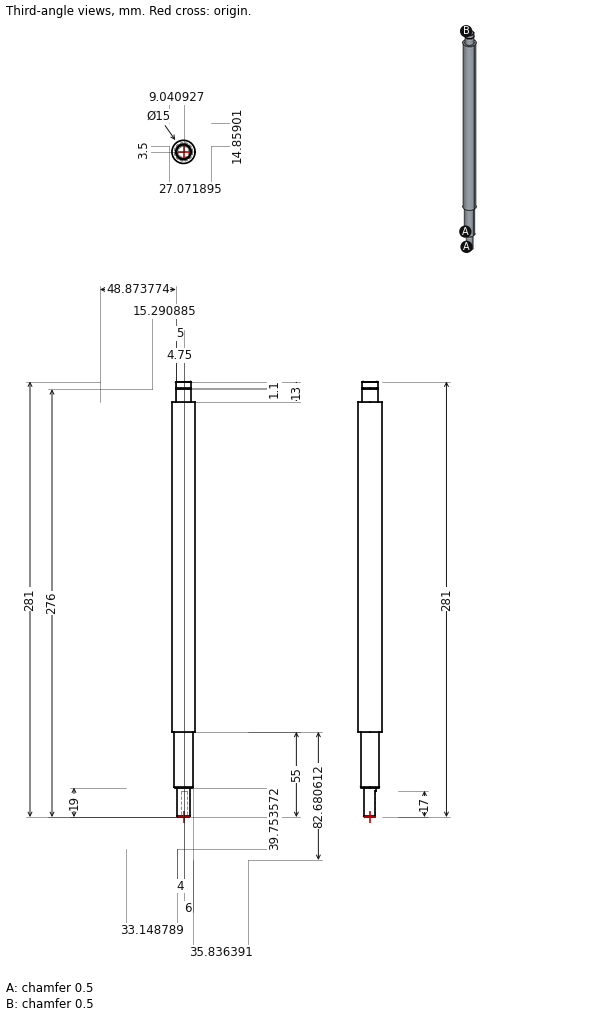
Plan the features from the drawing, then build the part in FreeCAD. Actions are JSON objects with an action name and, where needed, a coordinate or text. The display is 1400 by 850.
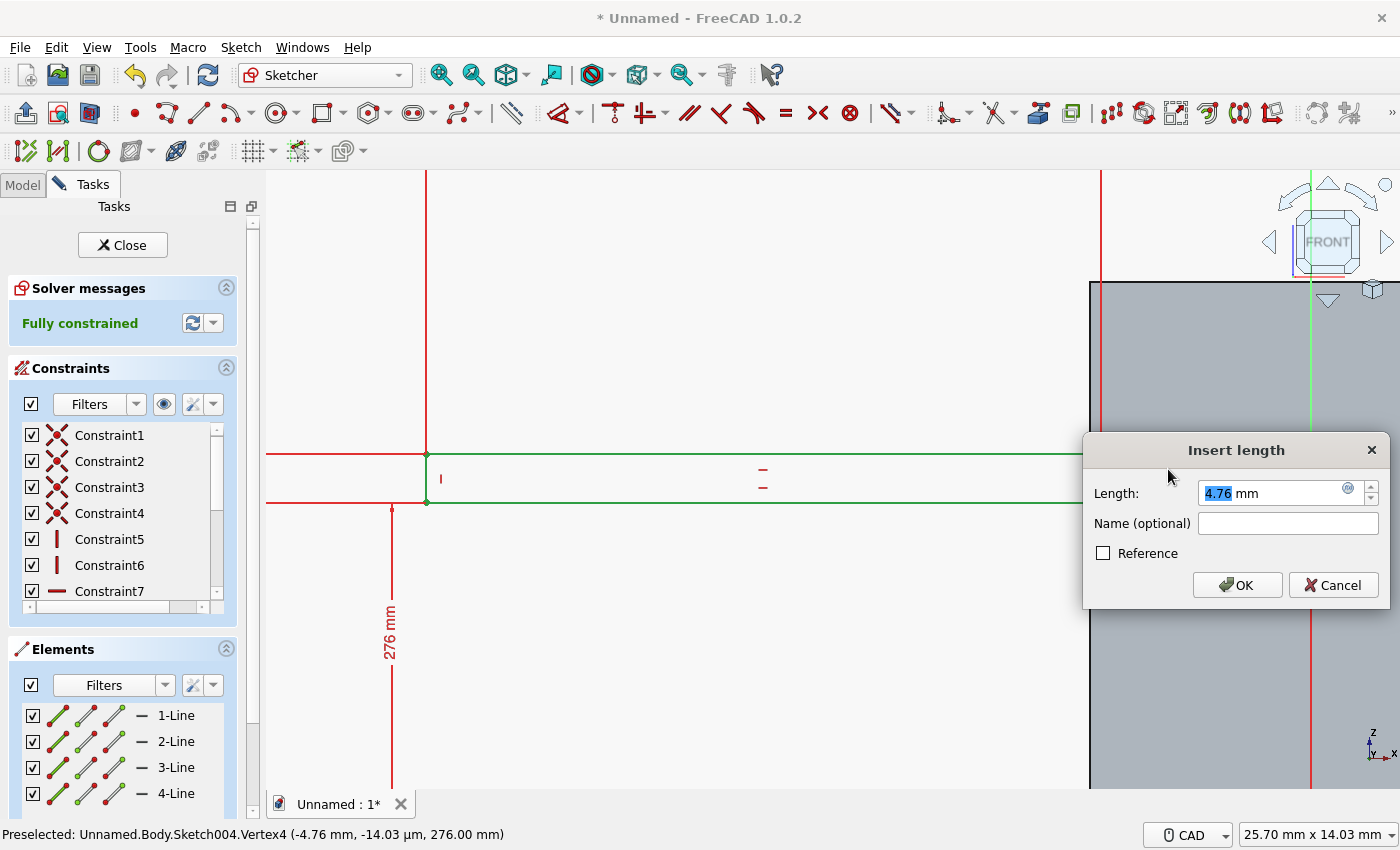
{"action": "type", "text": "4.75"}
{"action": "key", "text": "Return"}
{"action": "key", "text": "Escape"}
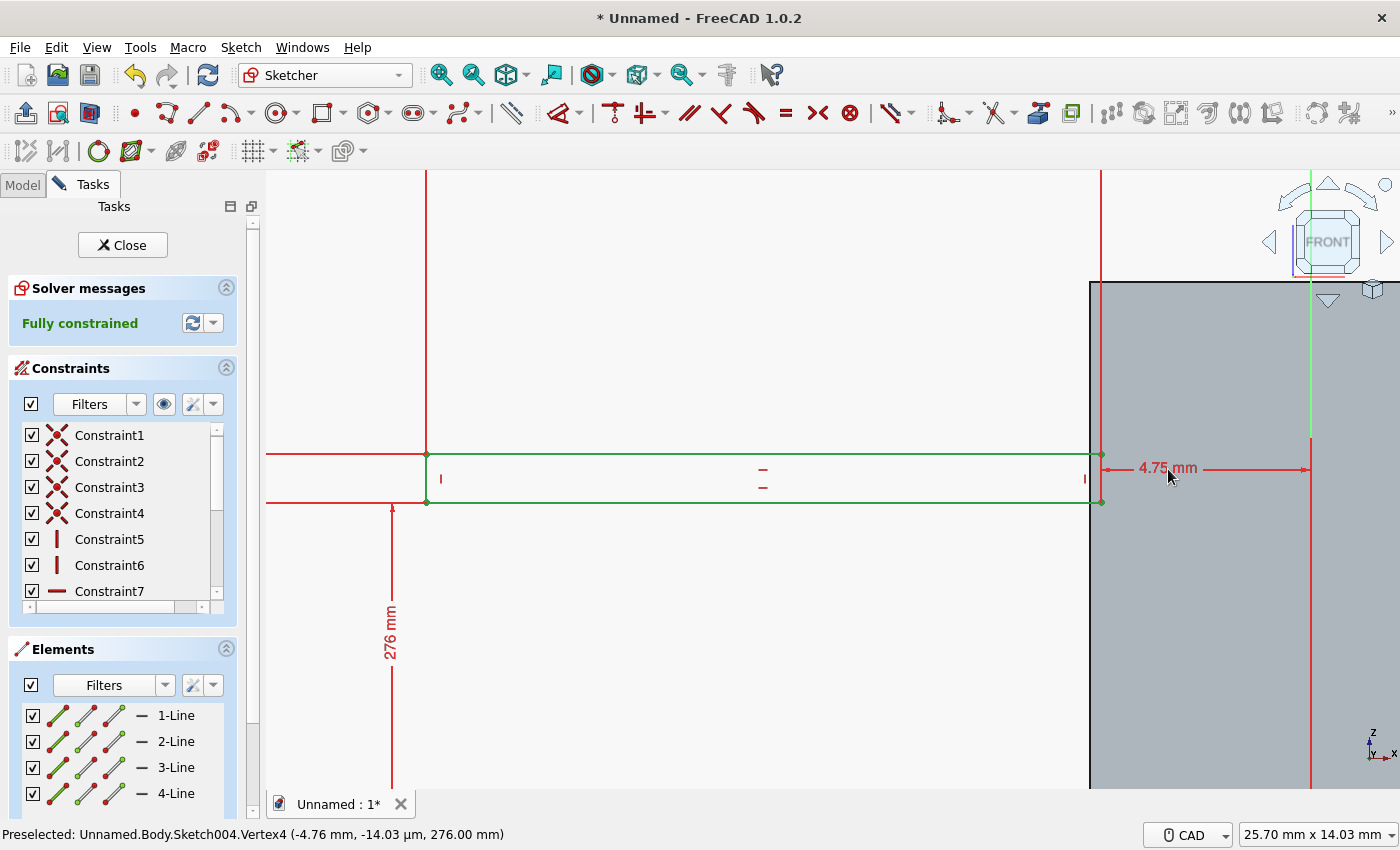
{"action": "left_click", "coordinate": [123, 245]}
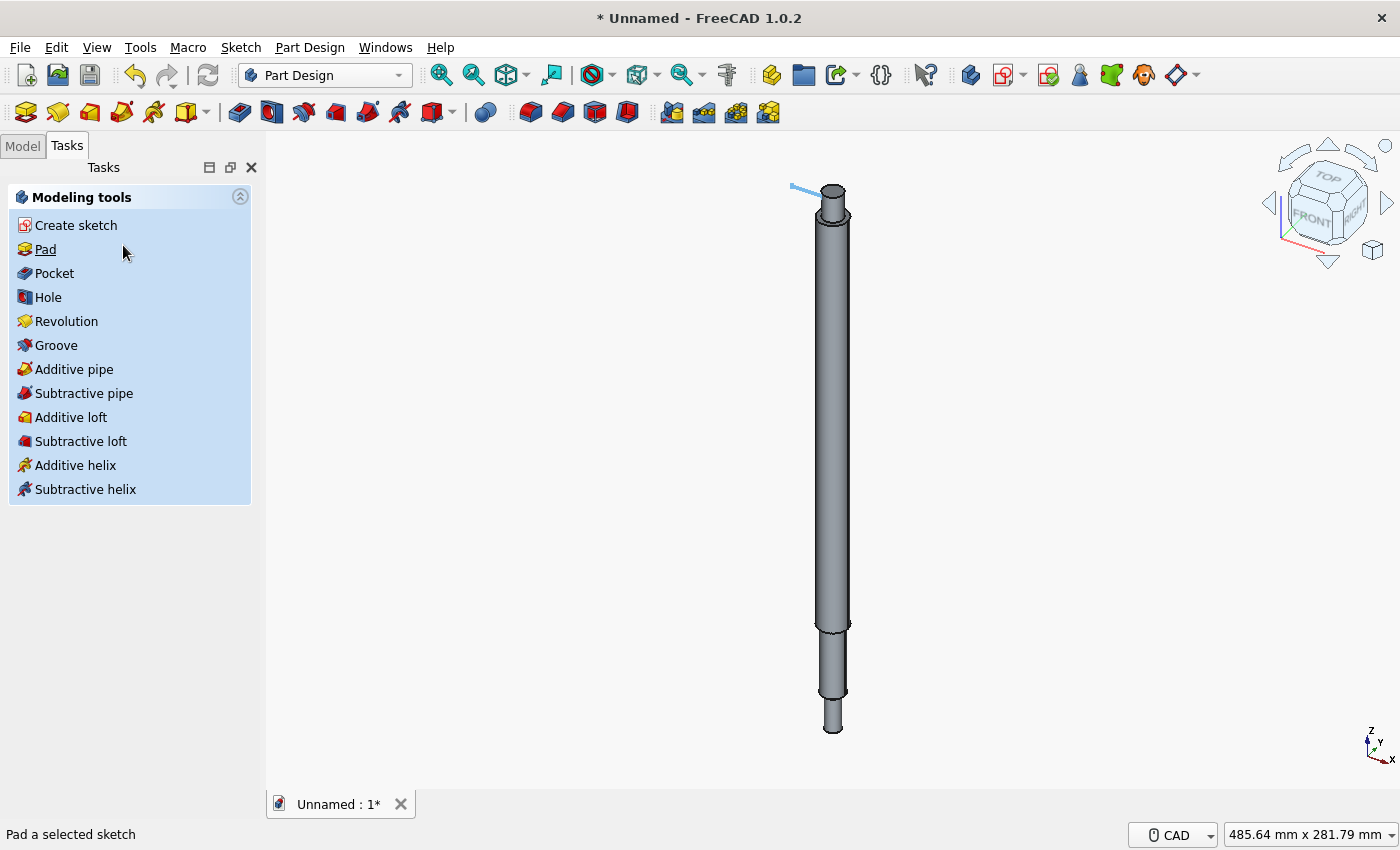
{"action": "left_click", "coordinate": [304, 112]}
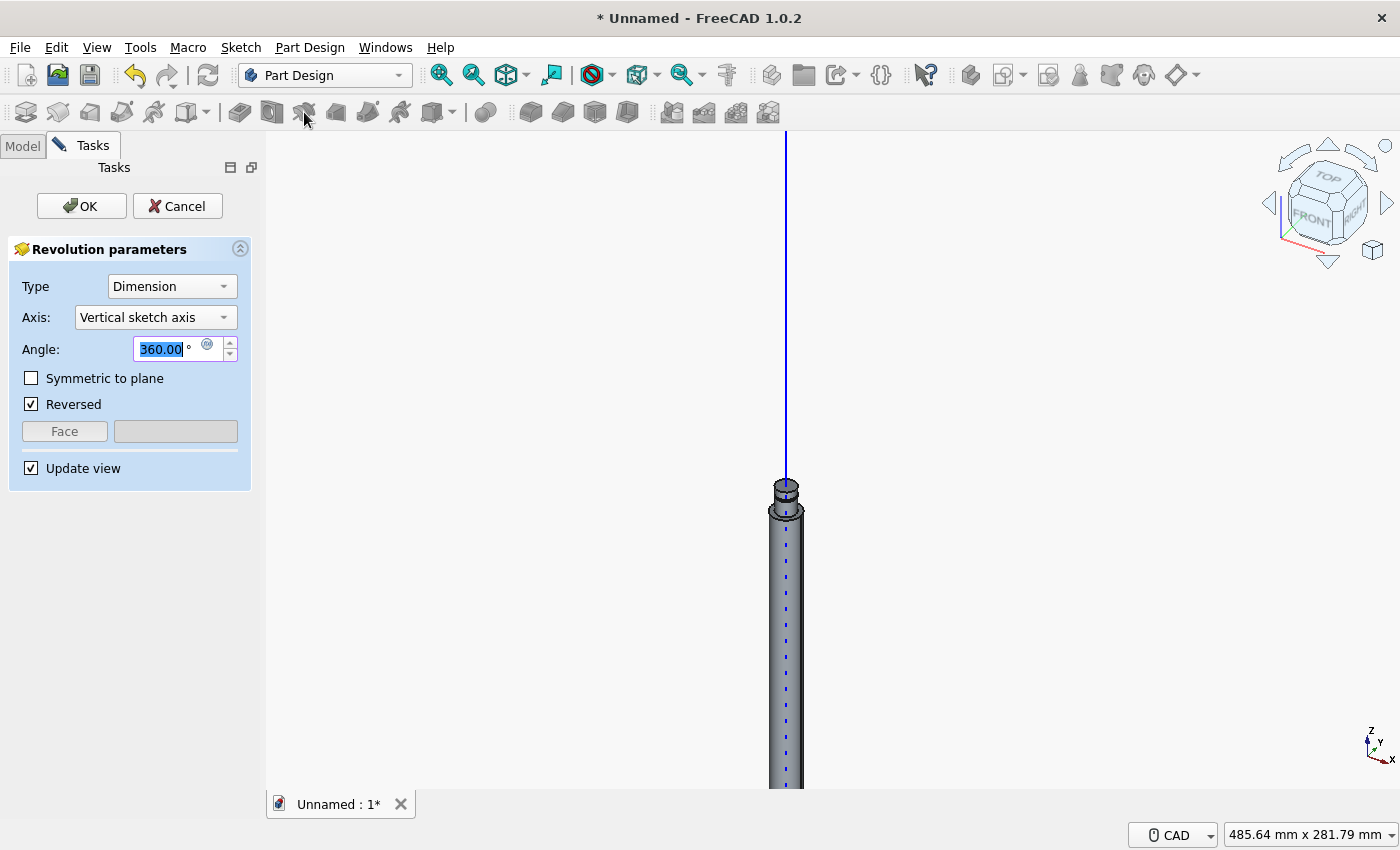
{"action": "left_click", "coordinate": [82, 206]}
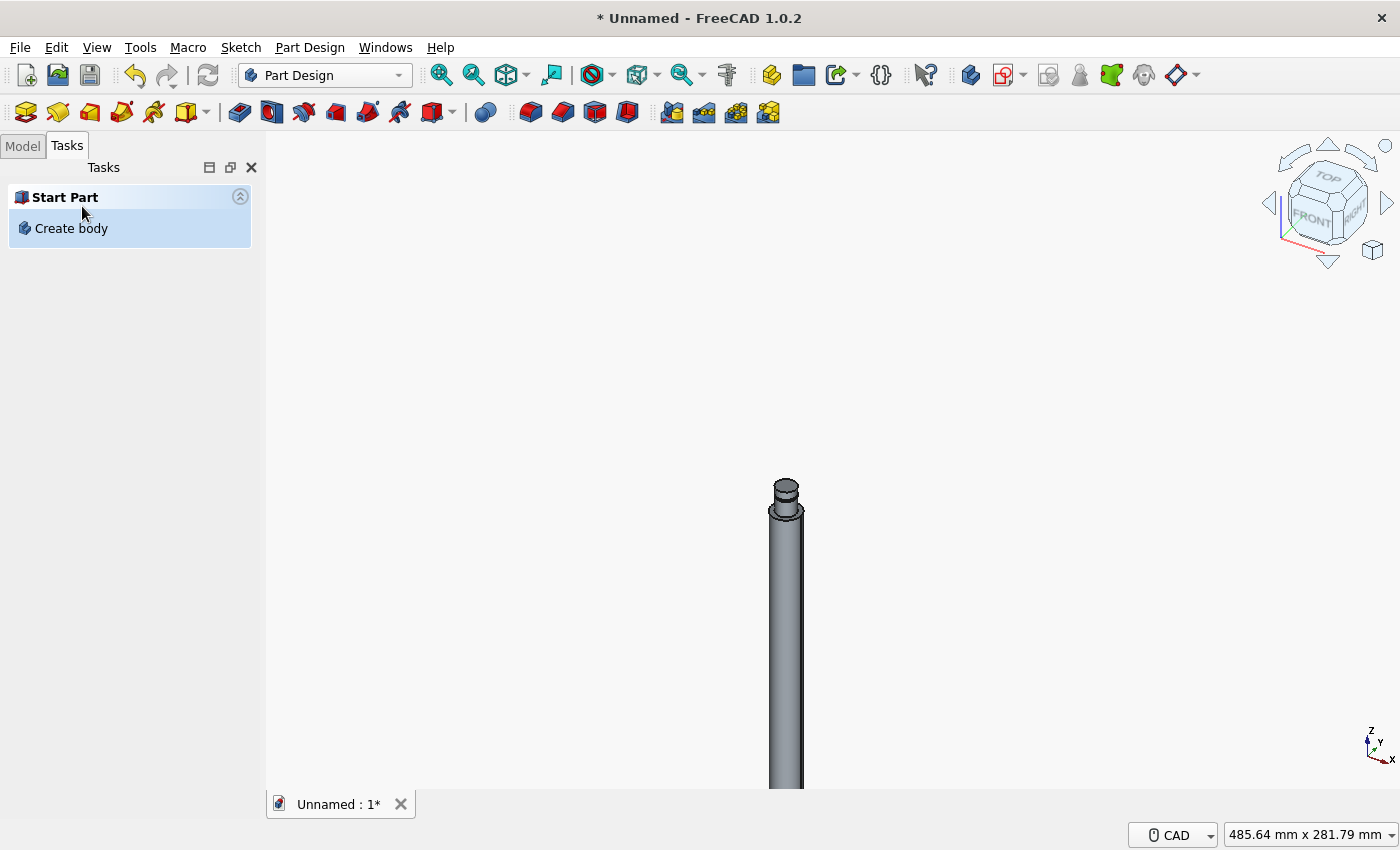
{"action": "left_click", "coordinate": [442, 76]}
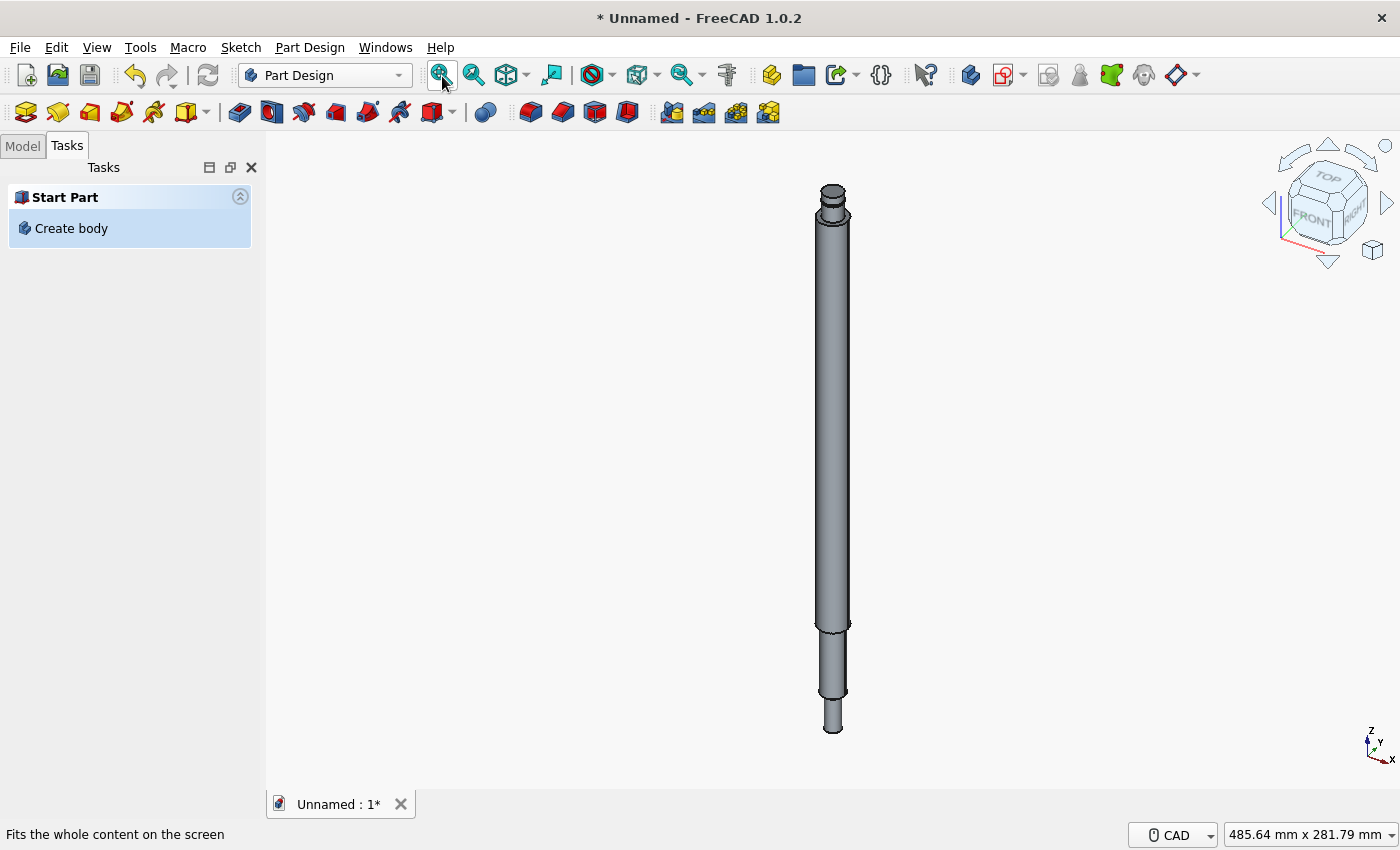
{"action": "left_click", "coordinate": [843, 194]}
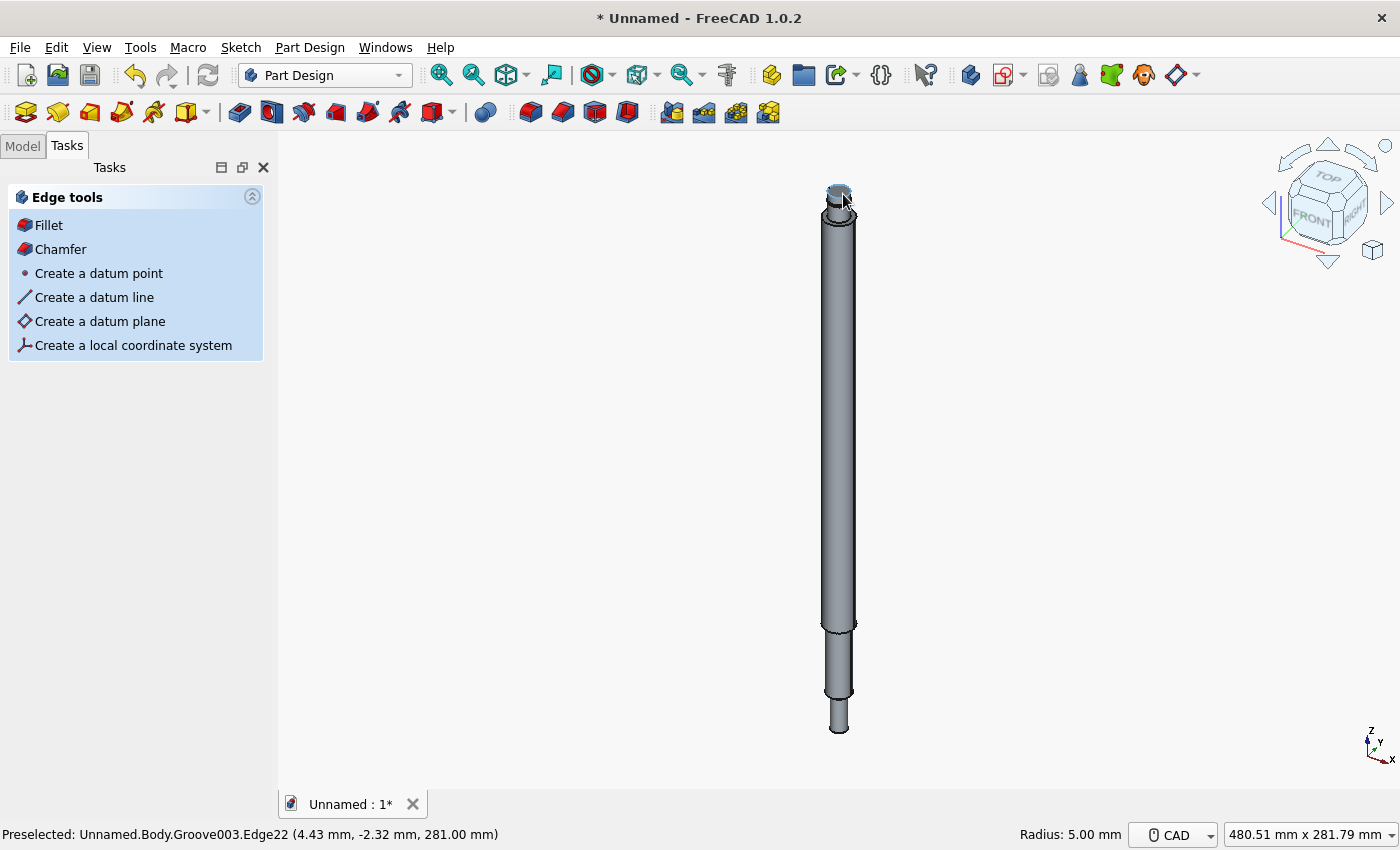
{"action": "left_click", "coordinate": [564, 112]}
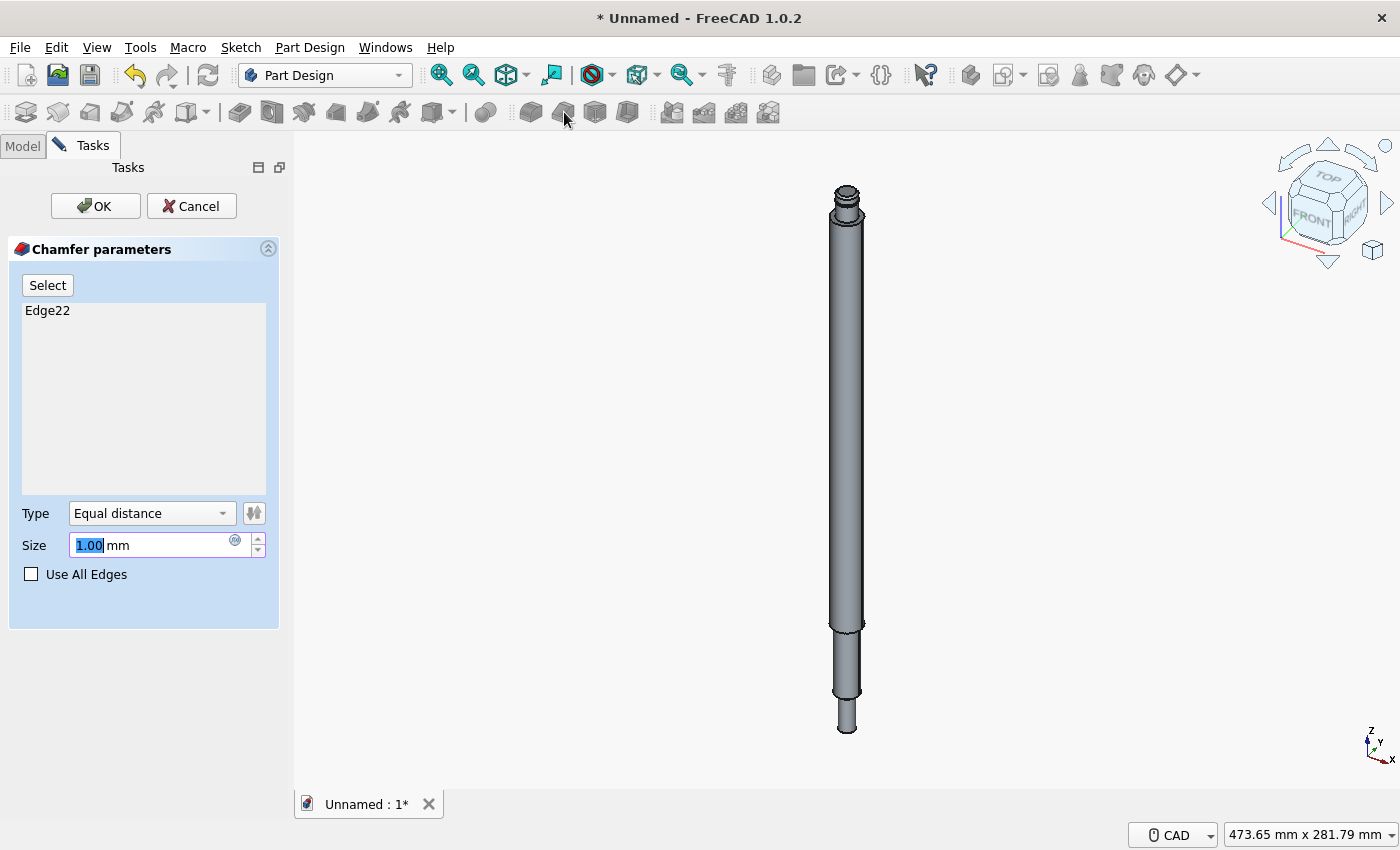
{"action": "type", "text": "0.5"}
{"action": "key", "text": "Tab"}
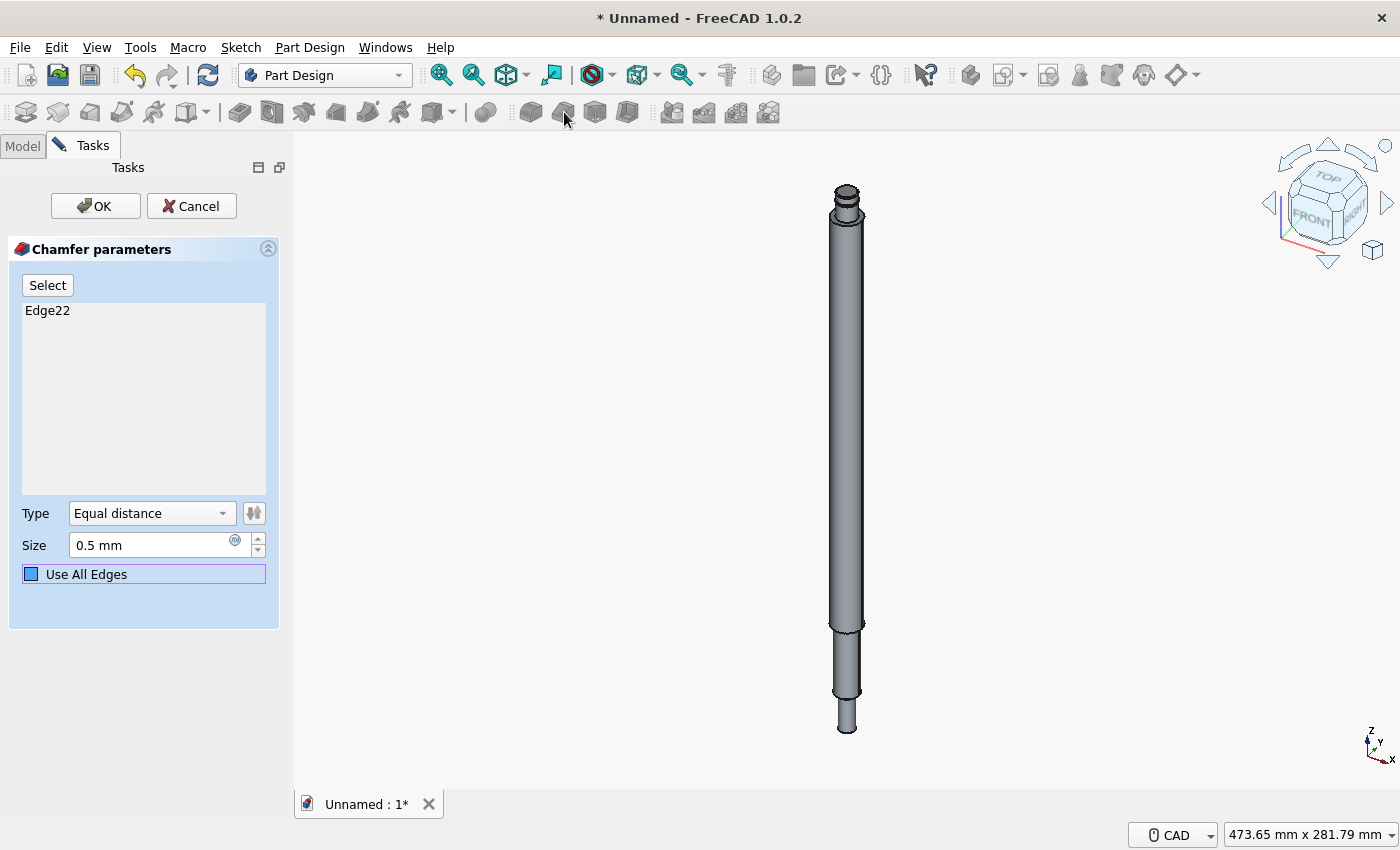
{"action": "left_click", "coordinate": [96, 206]}